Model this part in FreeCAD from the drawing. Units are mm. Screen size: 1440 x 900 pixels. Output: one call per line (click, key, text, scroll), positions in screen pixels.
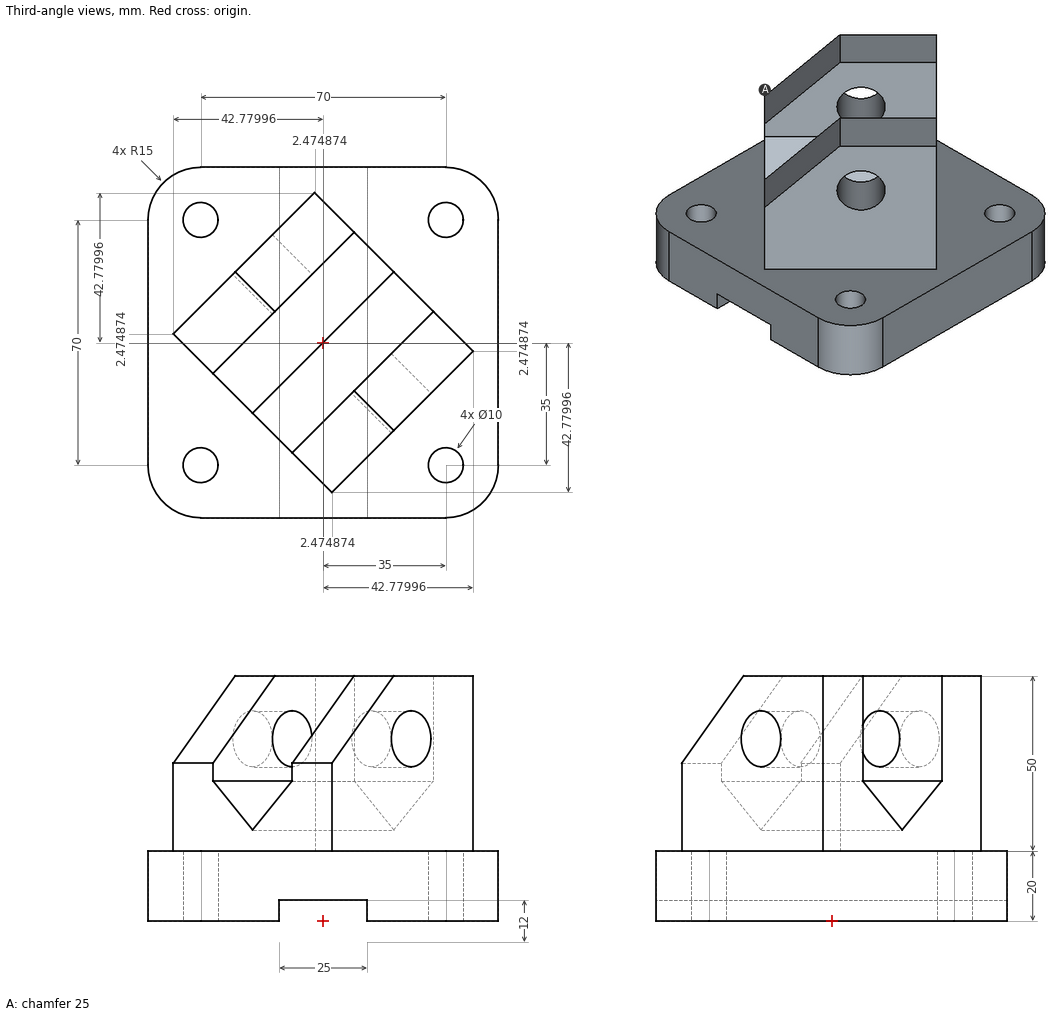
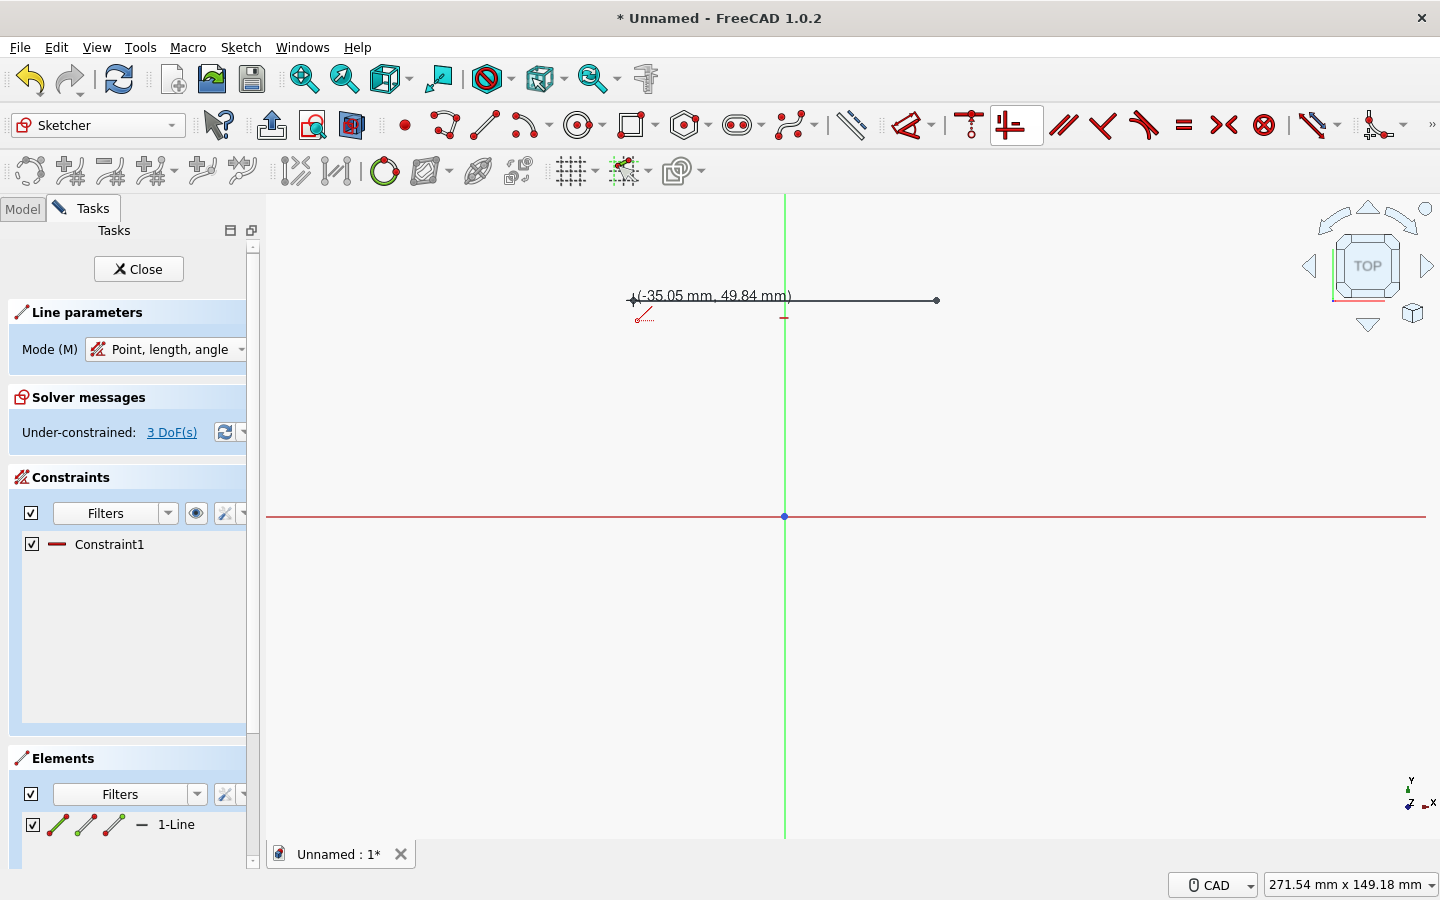
click(568, 365)
click(568, 668)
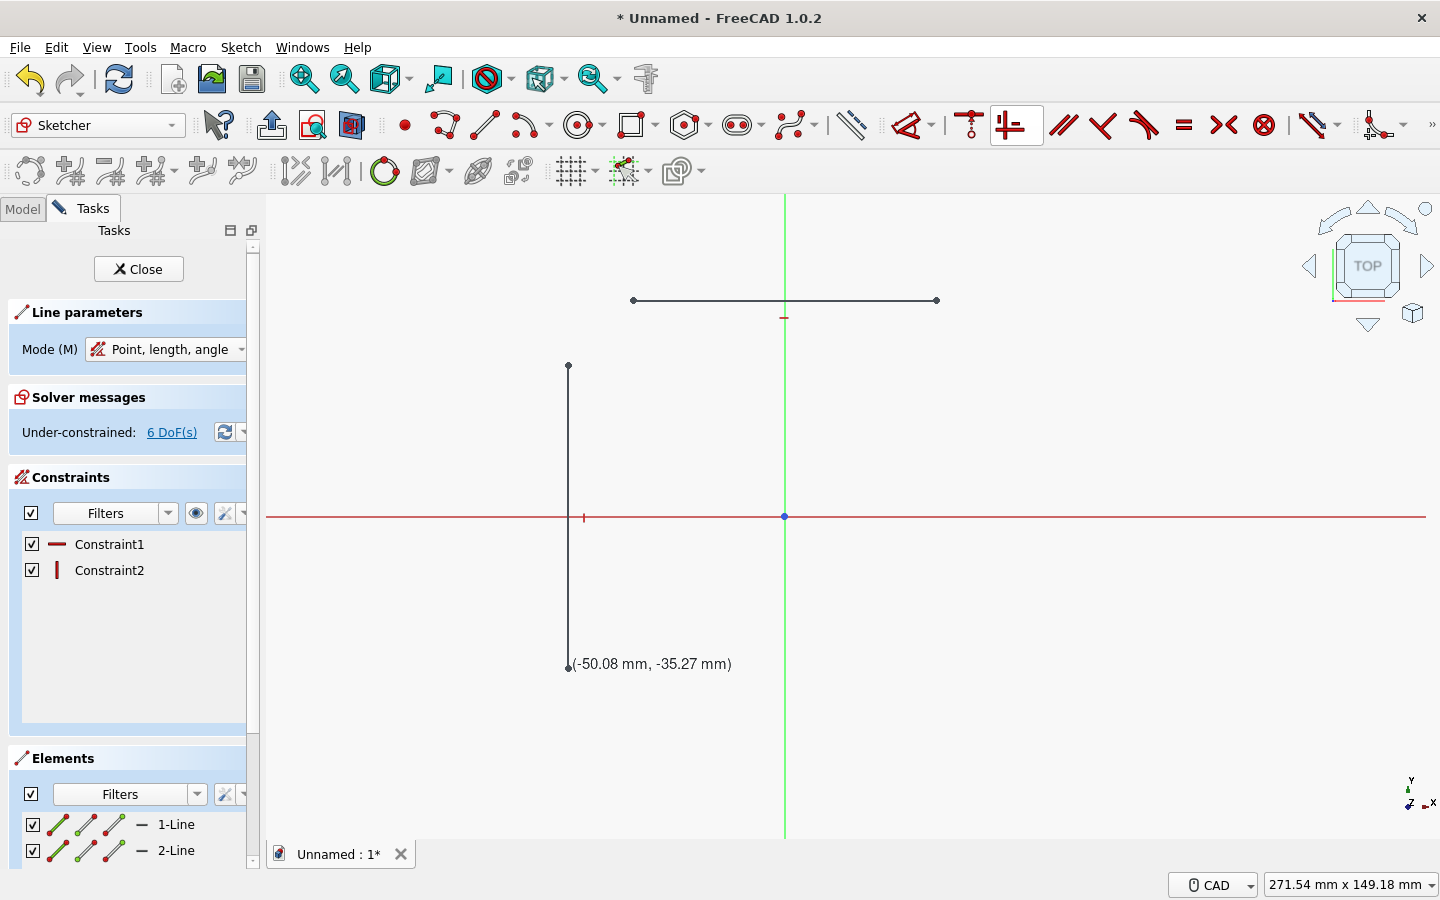
click(633, 733)
click(936, 733)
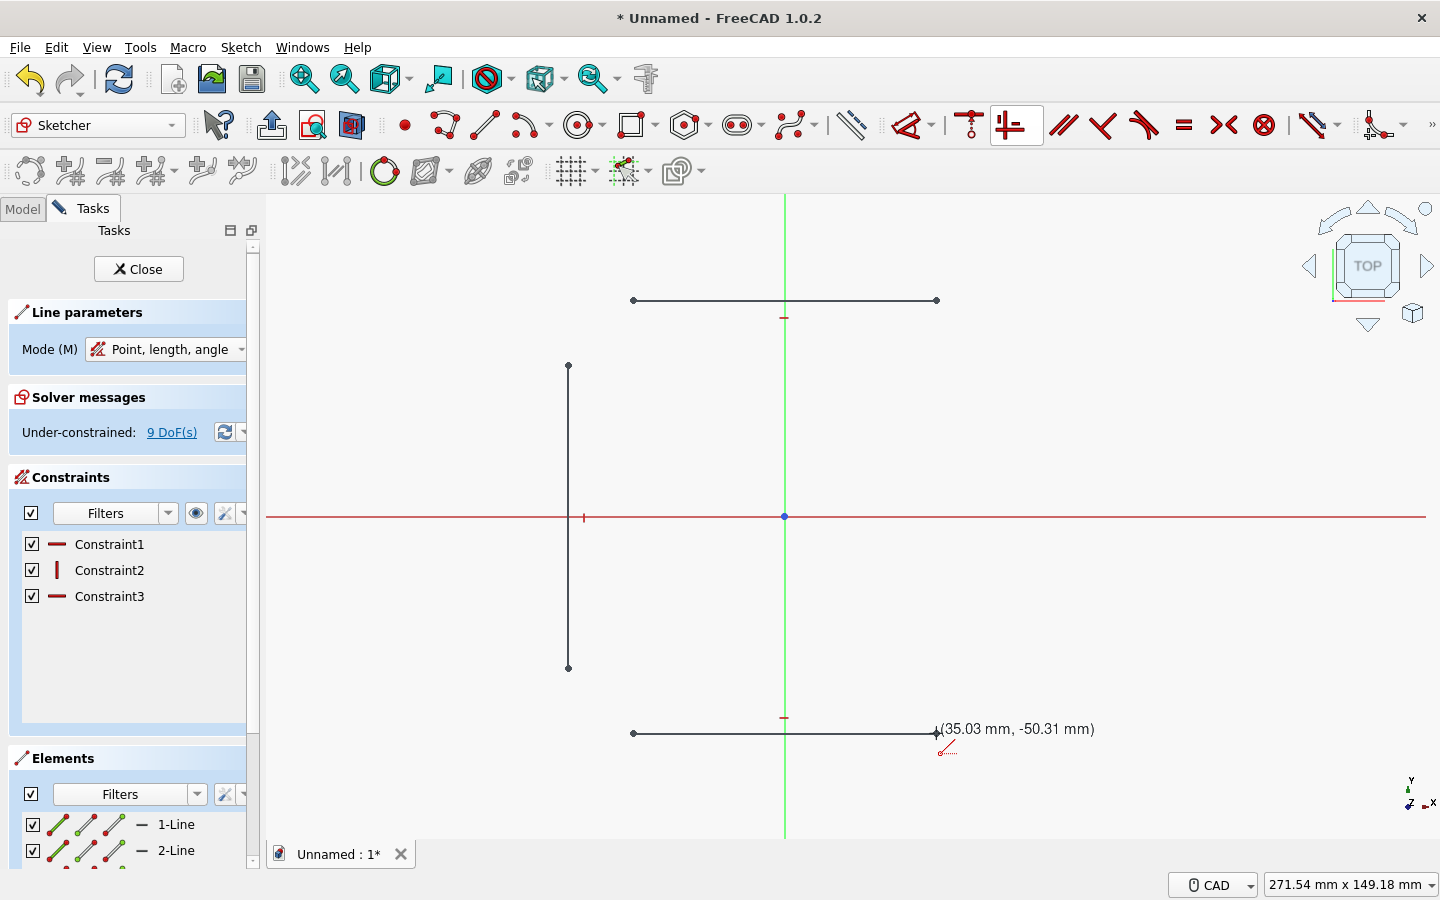
click(1001, 668)
click(1001, 365)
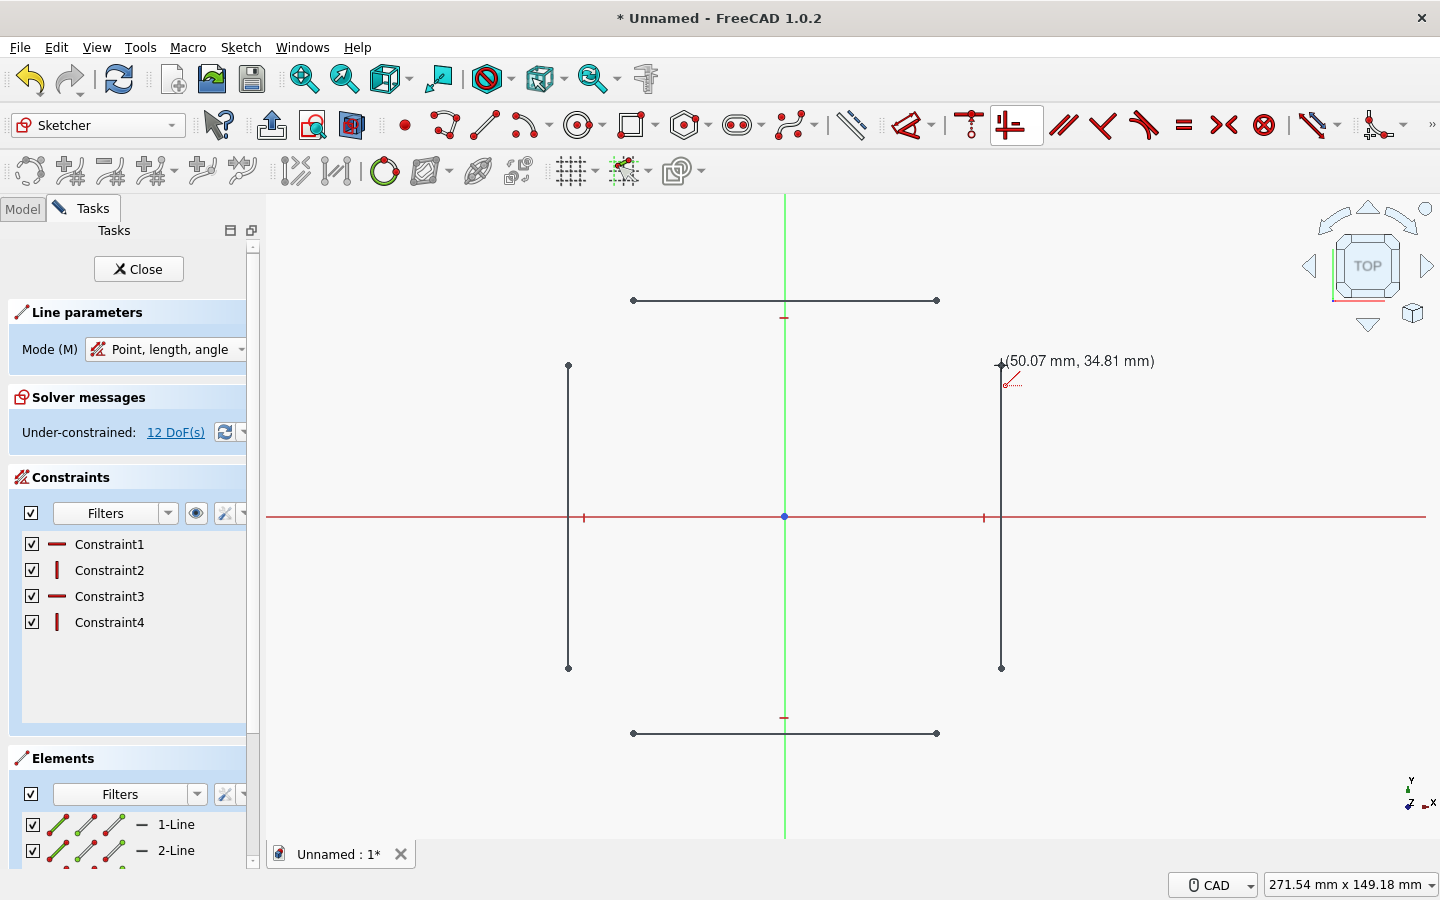
click(552, 126)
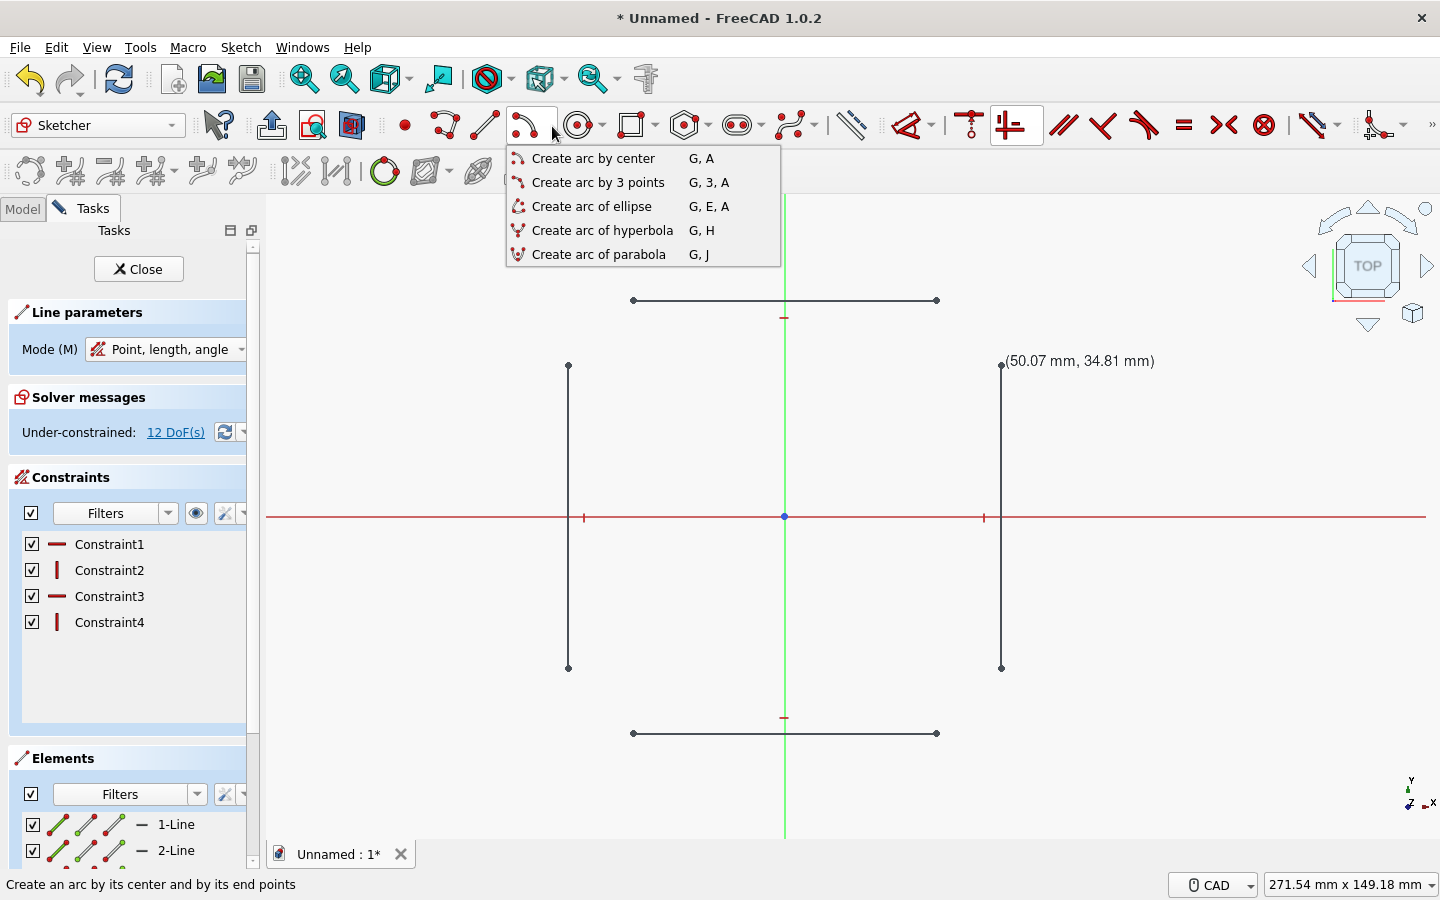
click(644, 182)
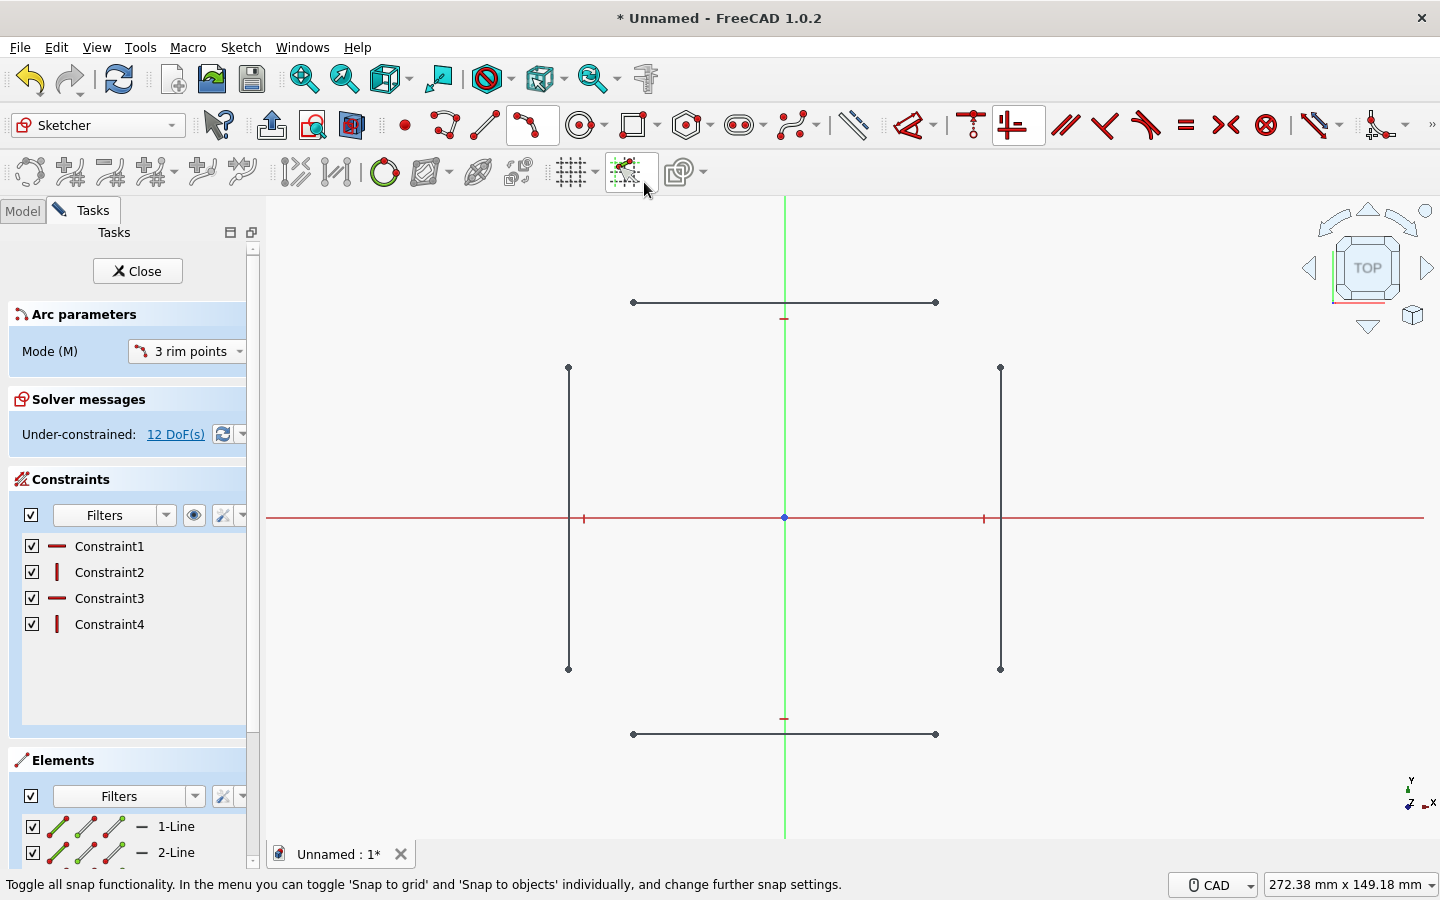
click(634, 303)
click(569, 367)
click(588, 321)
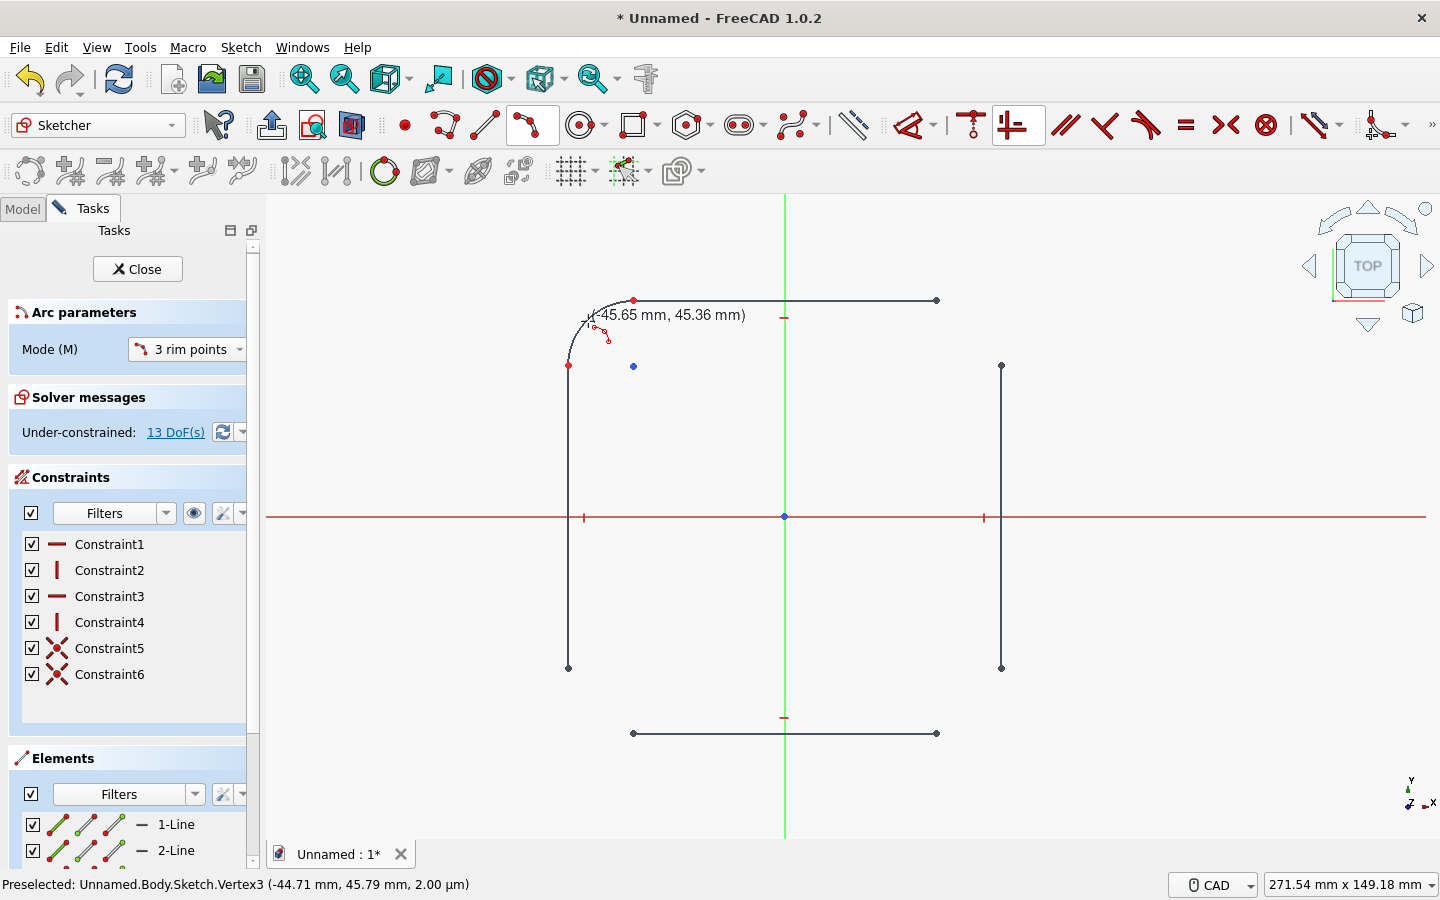
click(568, 669)
click(633, 734)
click(587, 714)